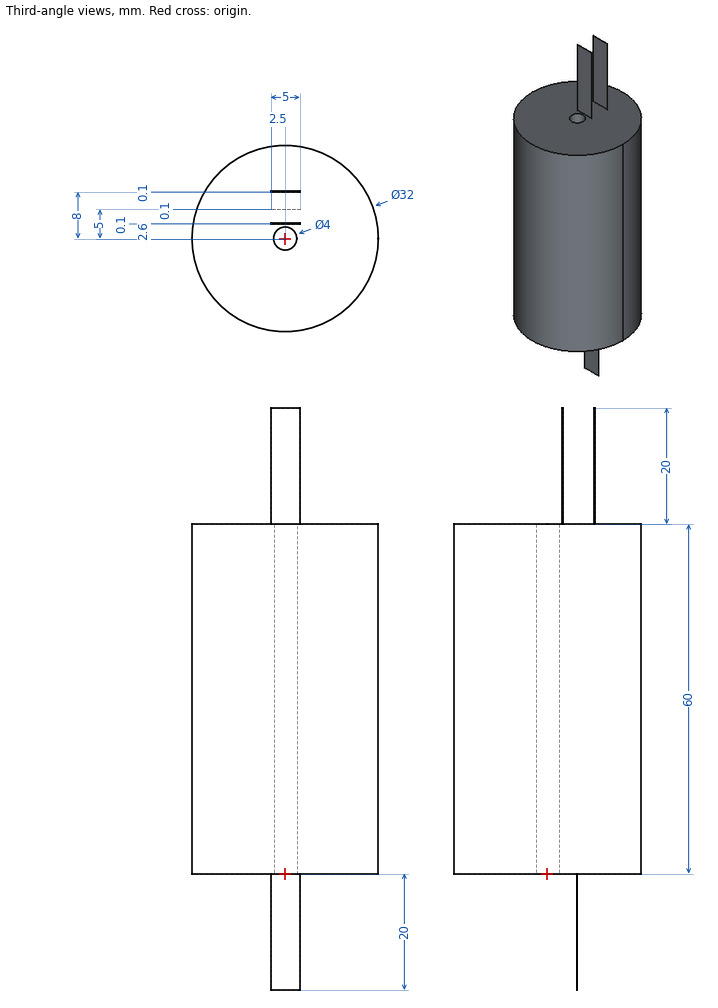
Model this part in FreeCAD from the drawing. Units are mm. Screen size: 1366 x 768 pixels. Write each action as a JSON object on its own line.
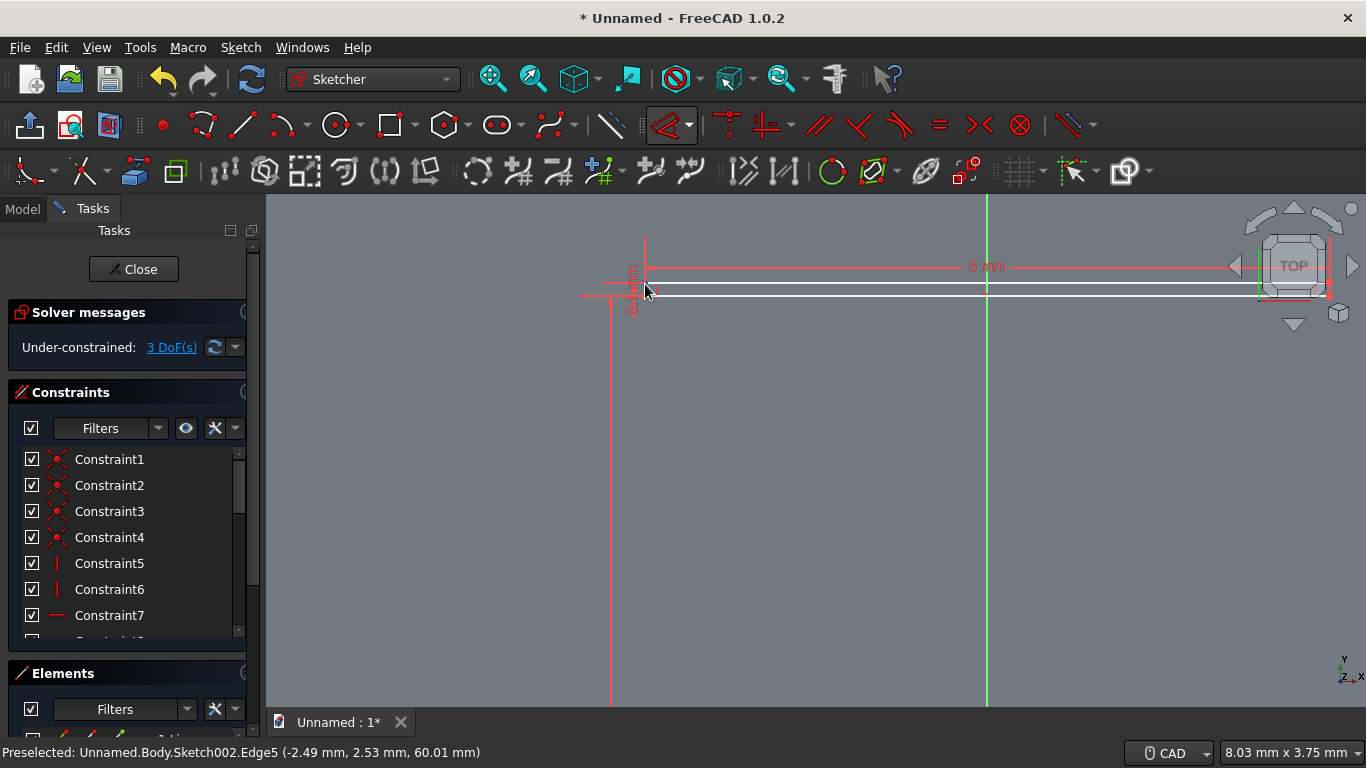
{"action": "left_click", "coordinate": [645, 283]}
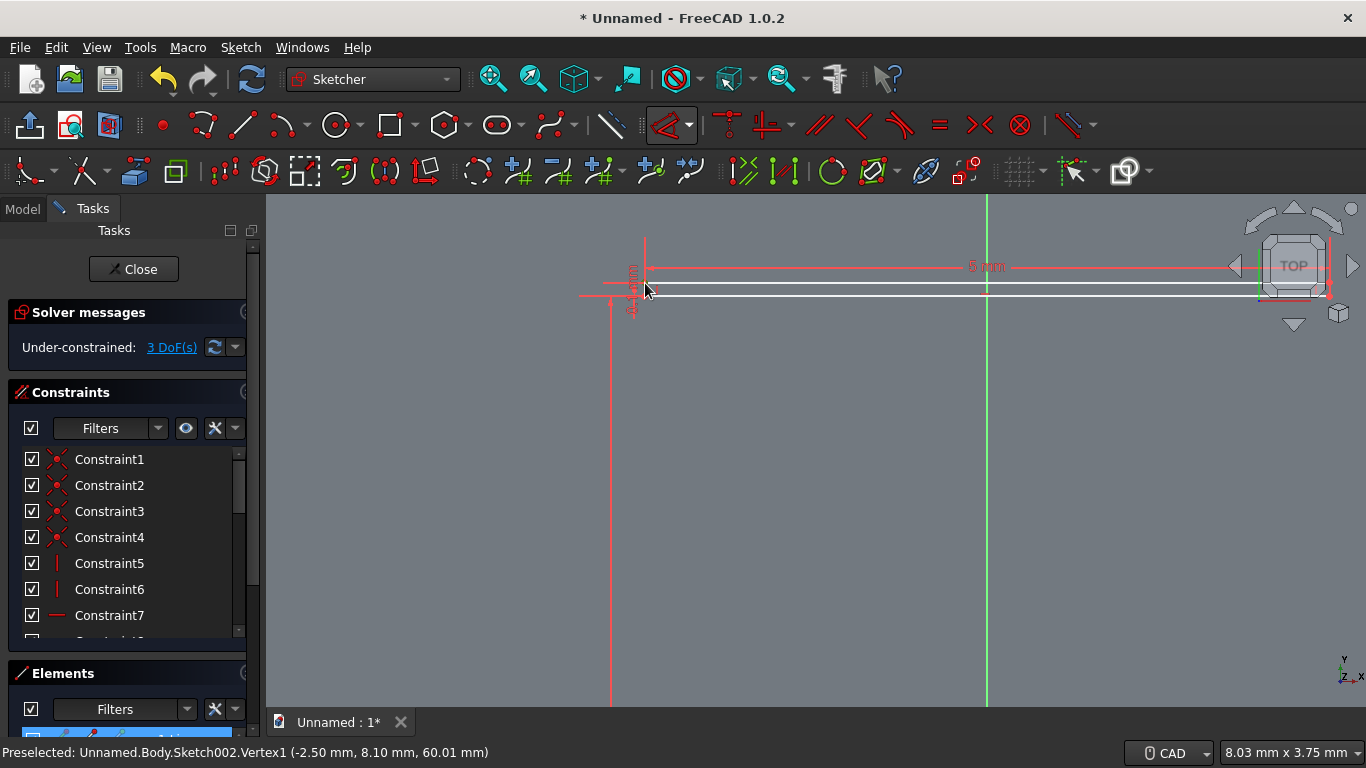
{"action": "key", "text": "l"}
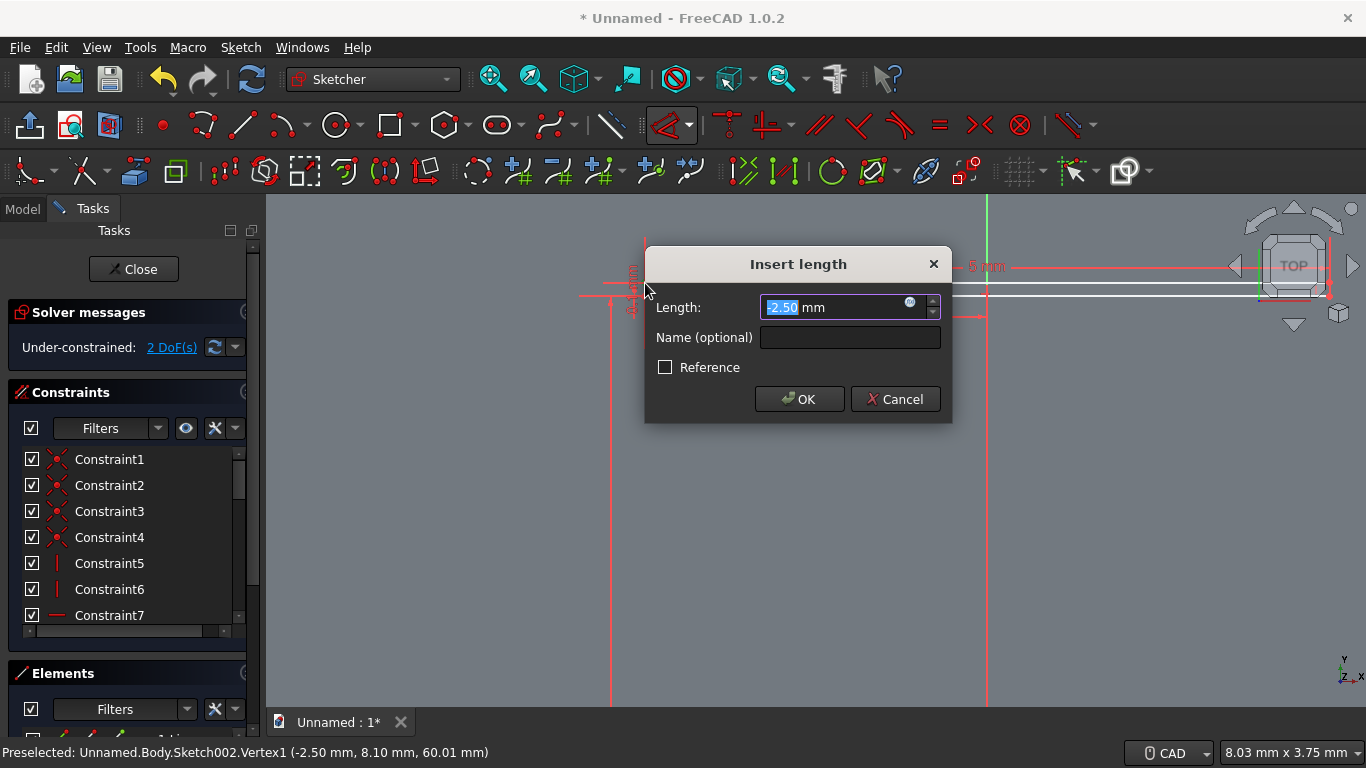
{"action": "type", "text": "-2.5"}
{"action": "key", "text": "Return"}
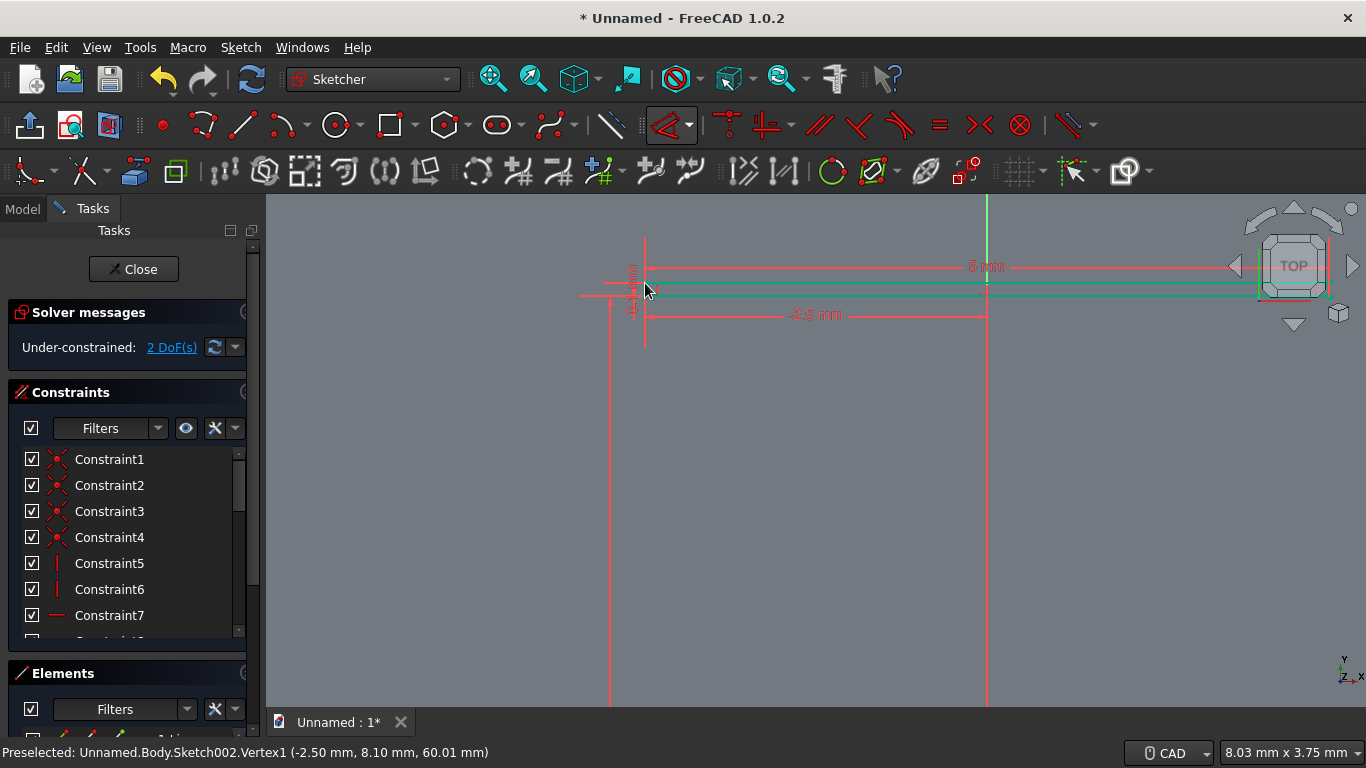
{"action": "scroll", "coordinate": [644, 284], "scroll_direction": "down", "scroll_amount": 6}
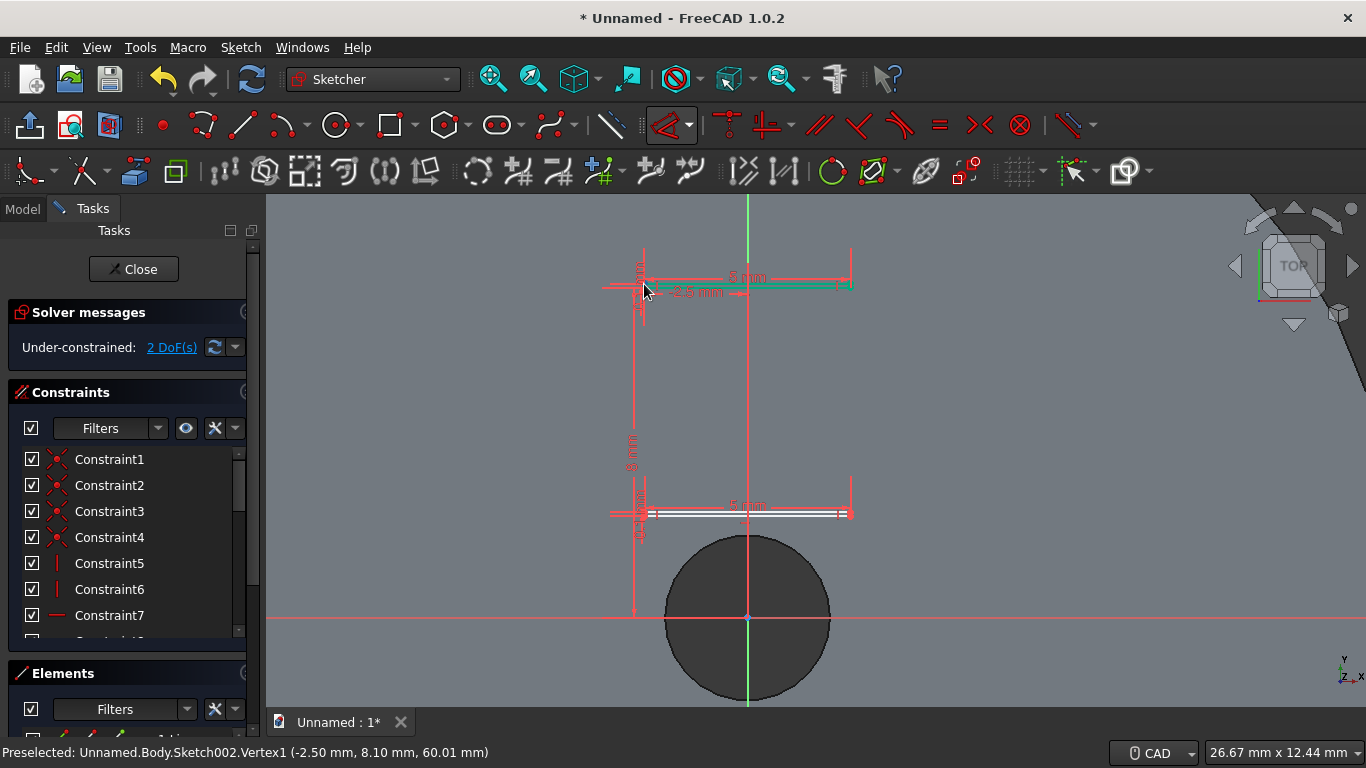
{"action": "scroll", "coordinate": [645, 512], "scroll_direction": "up", "scroll_amount": 6}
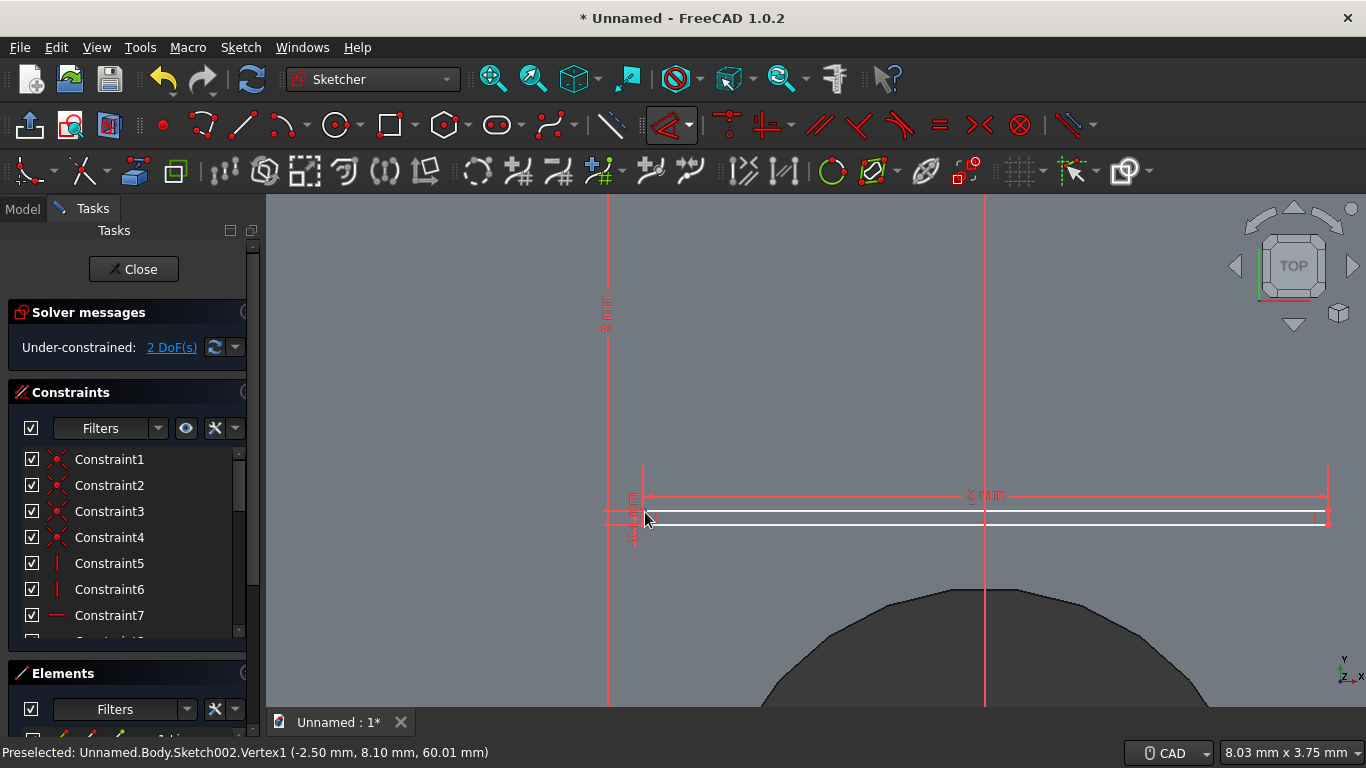
{"action": "left_click", "coordinate": [643, 511]}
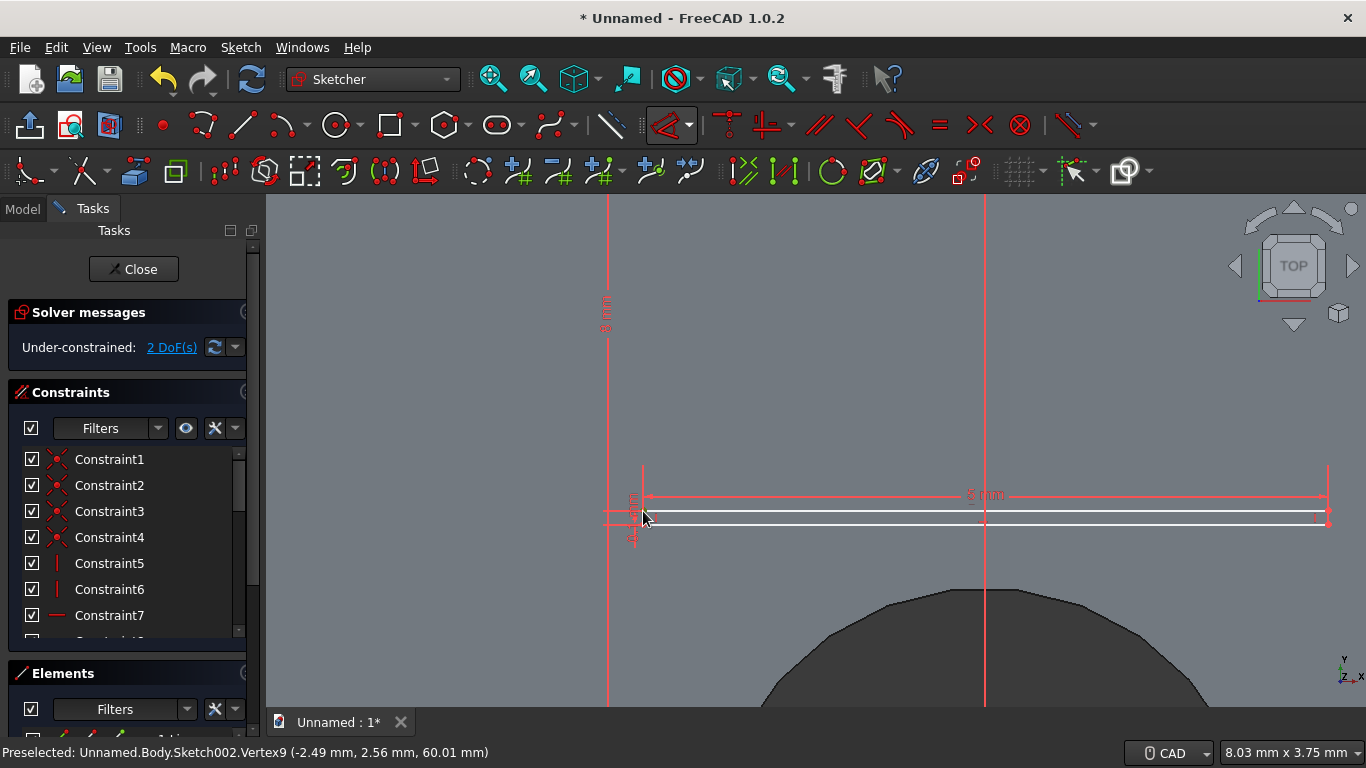
{"action": "key", "text": "l"}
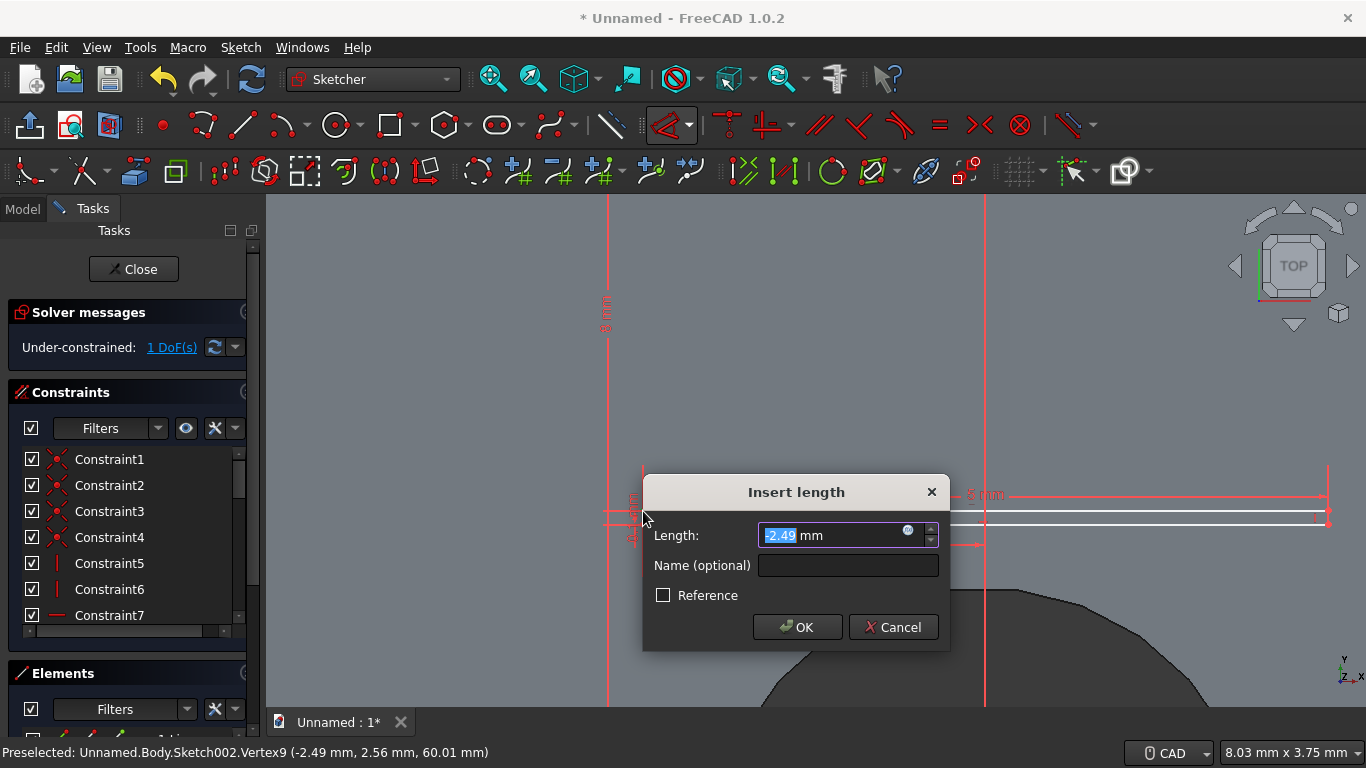
{"action": "type", "text": "-2.5"}
{"action": "key", "text": "Return"}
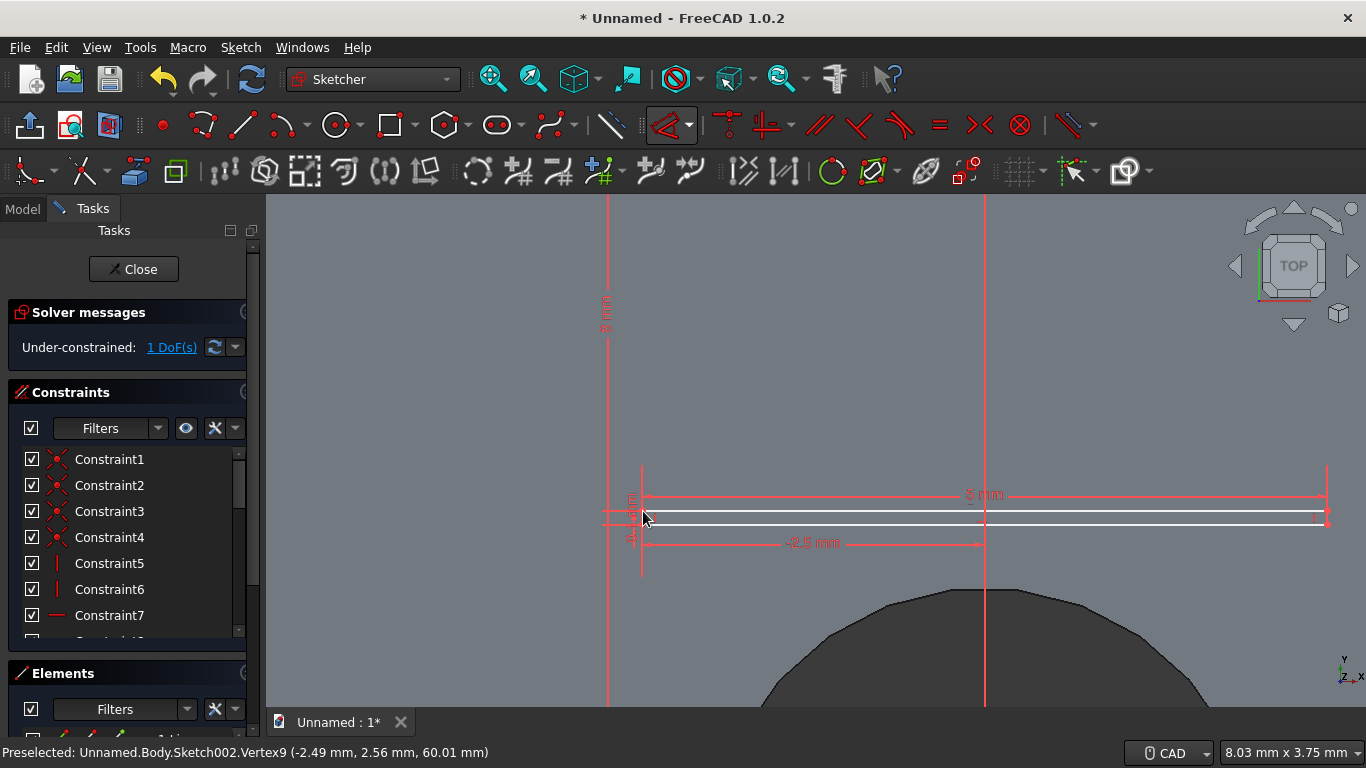
{"action": "left_click", "coordinate": [642, 511]}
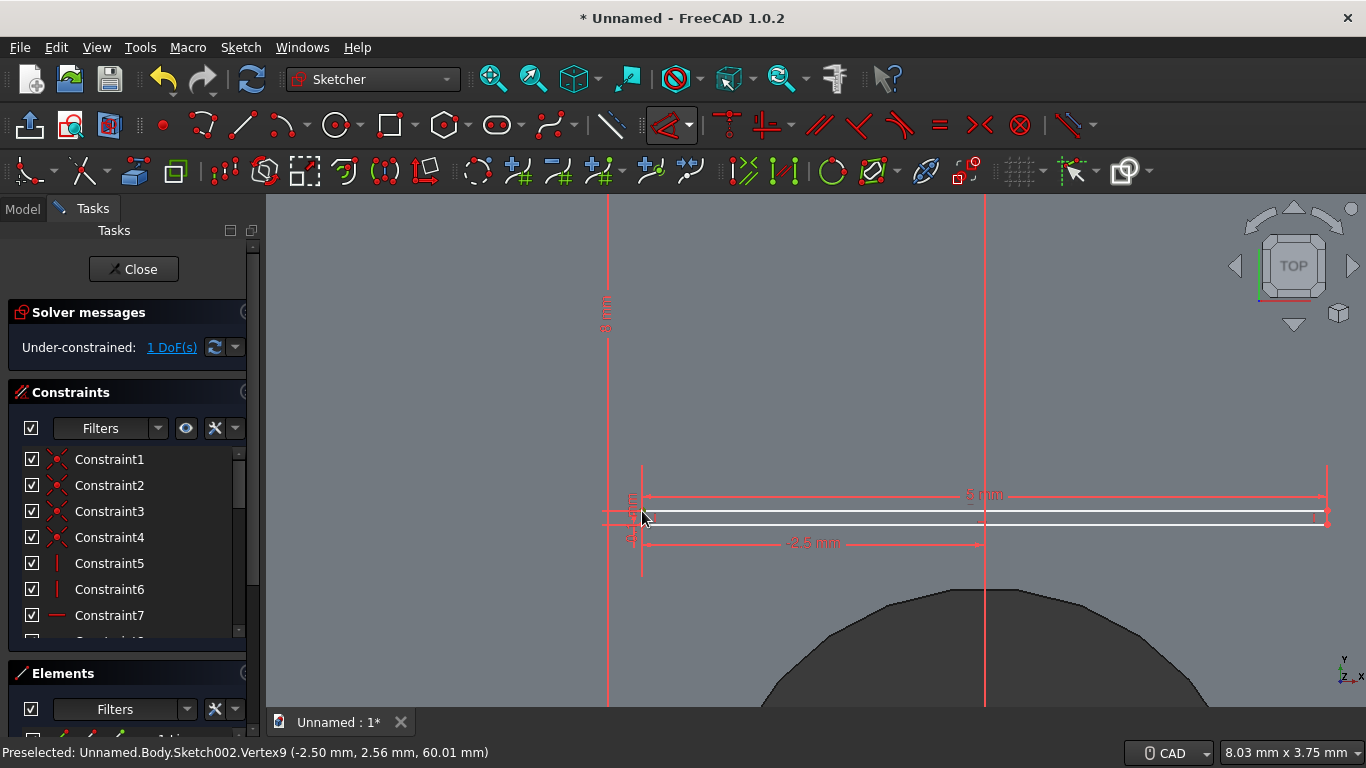
{"action": "left_click", "coordinate": [692, 126]}